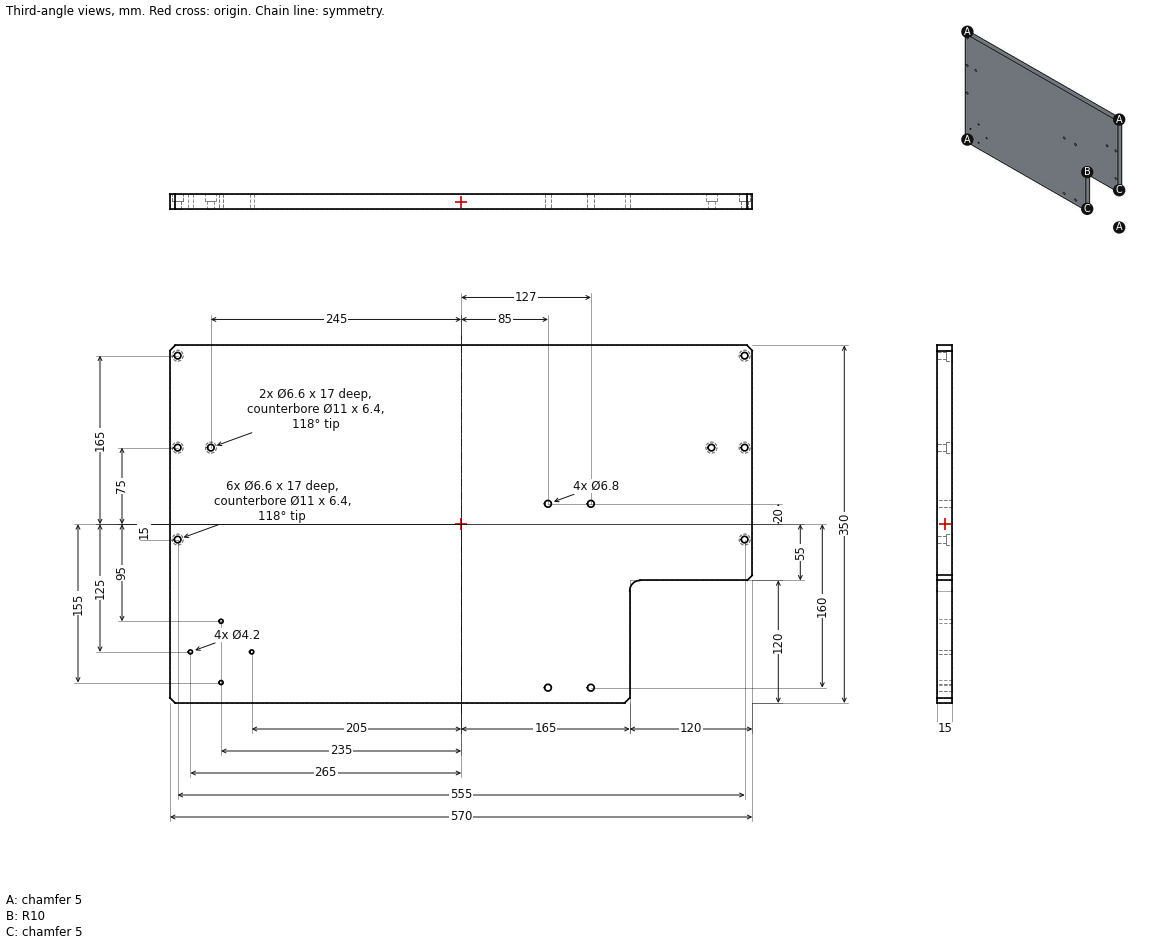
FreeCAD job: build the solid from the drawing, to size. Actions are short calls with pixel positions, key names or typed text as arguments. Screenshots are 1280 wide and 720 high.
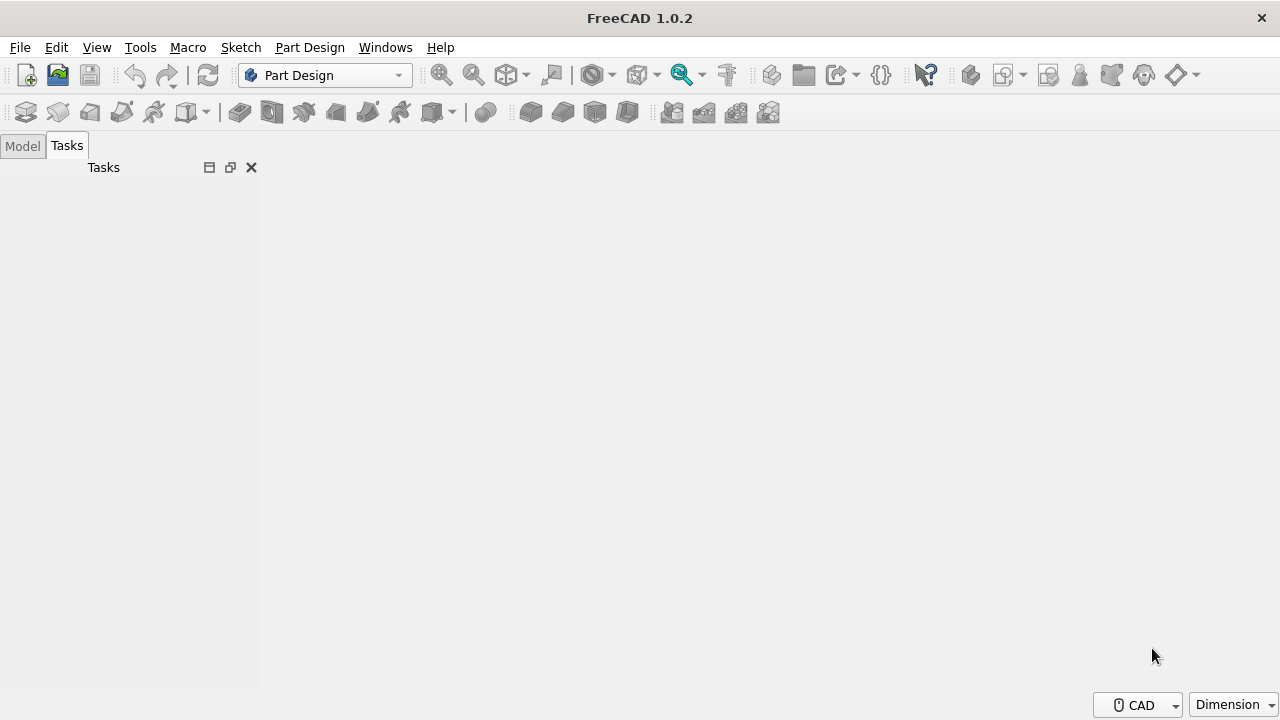
click(26, 76)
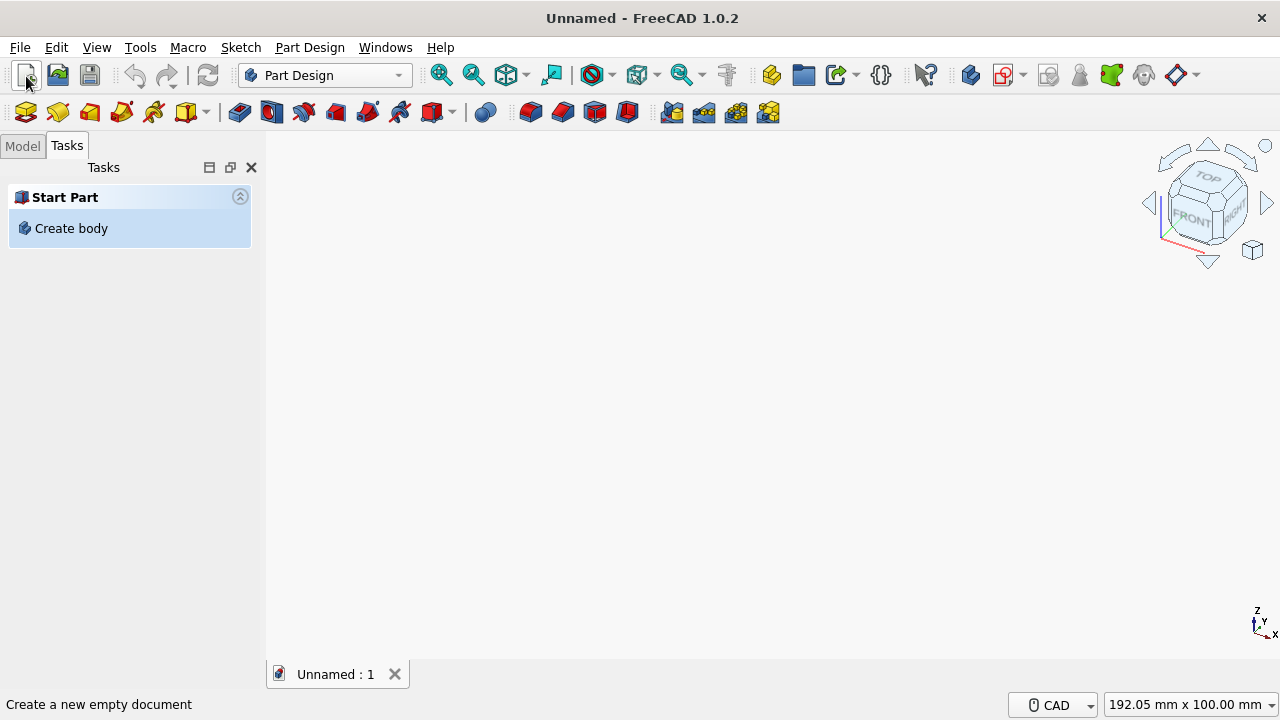
click(1004, 76)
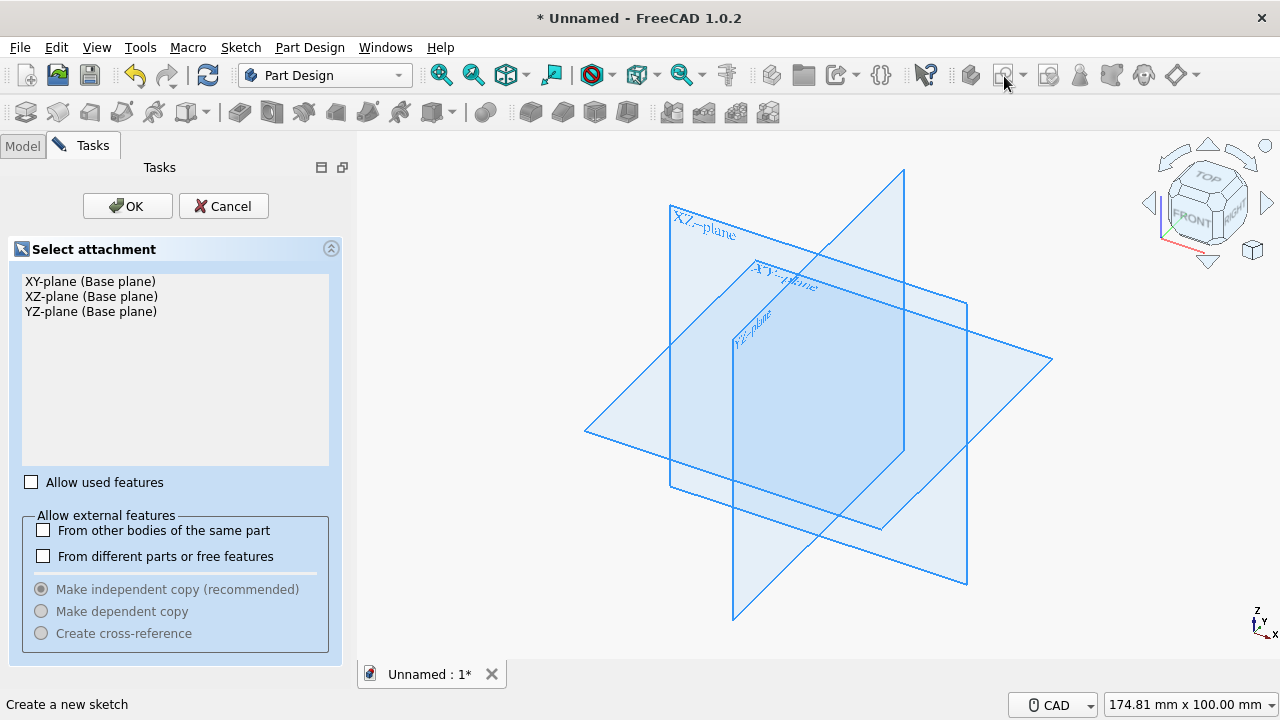
click(82, 296)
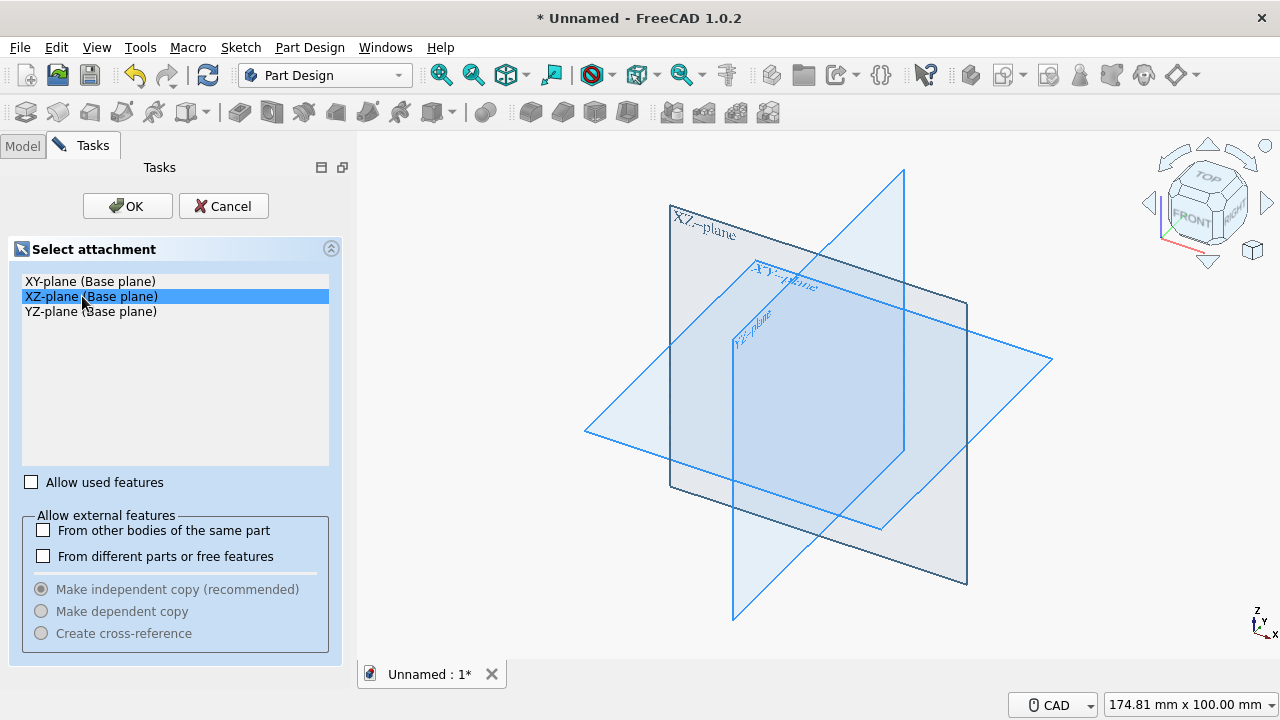
click(128, 206)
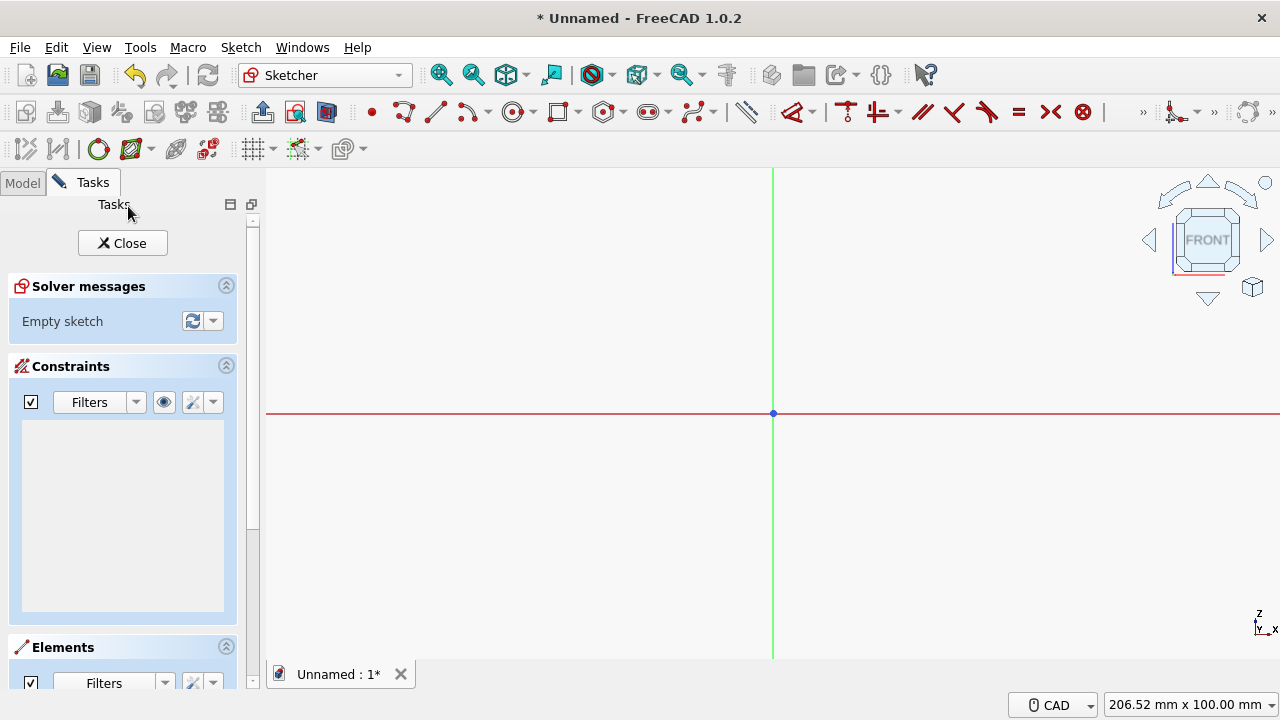
scroll(691, 414, down, 9)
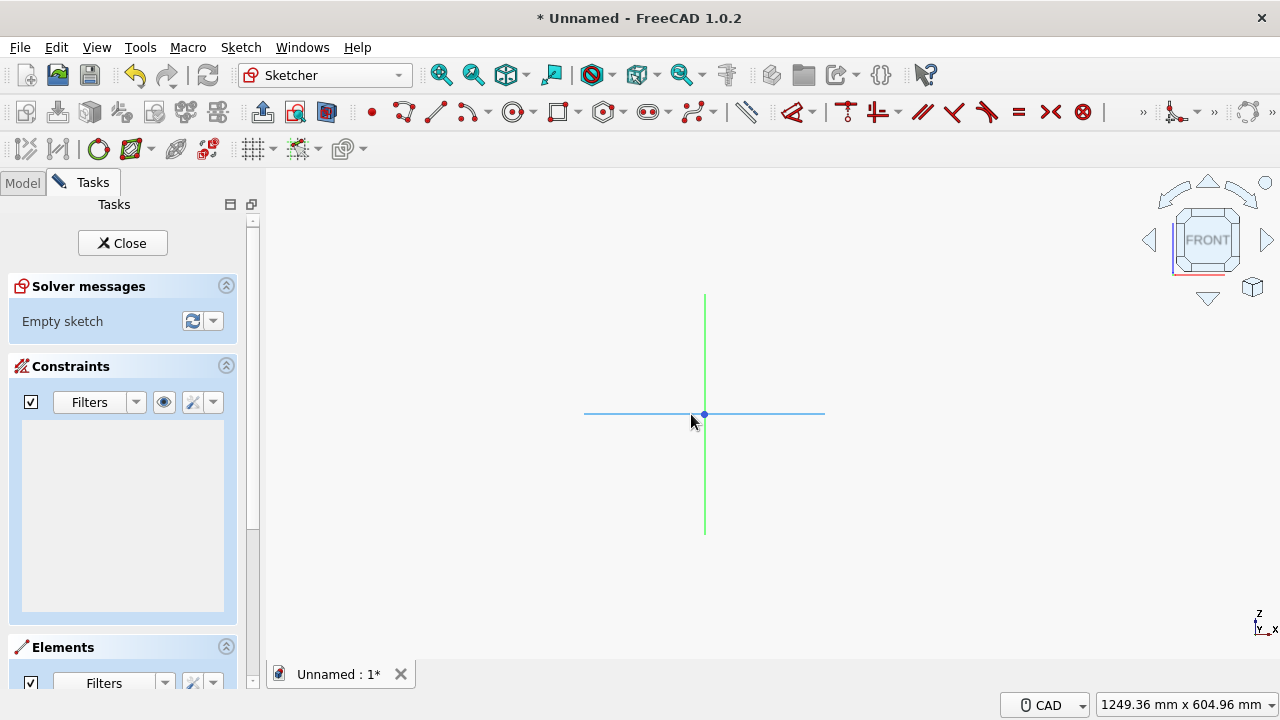
click(580, 112)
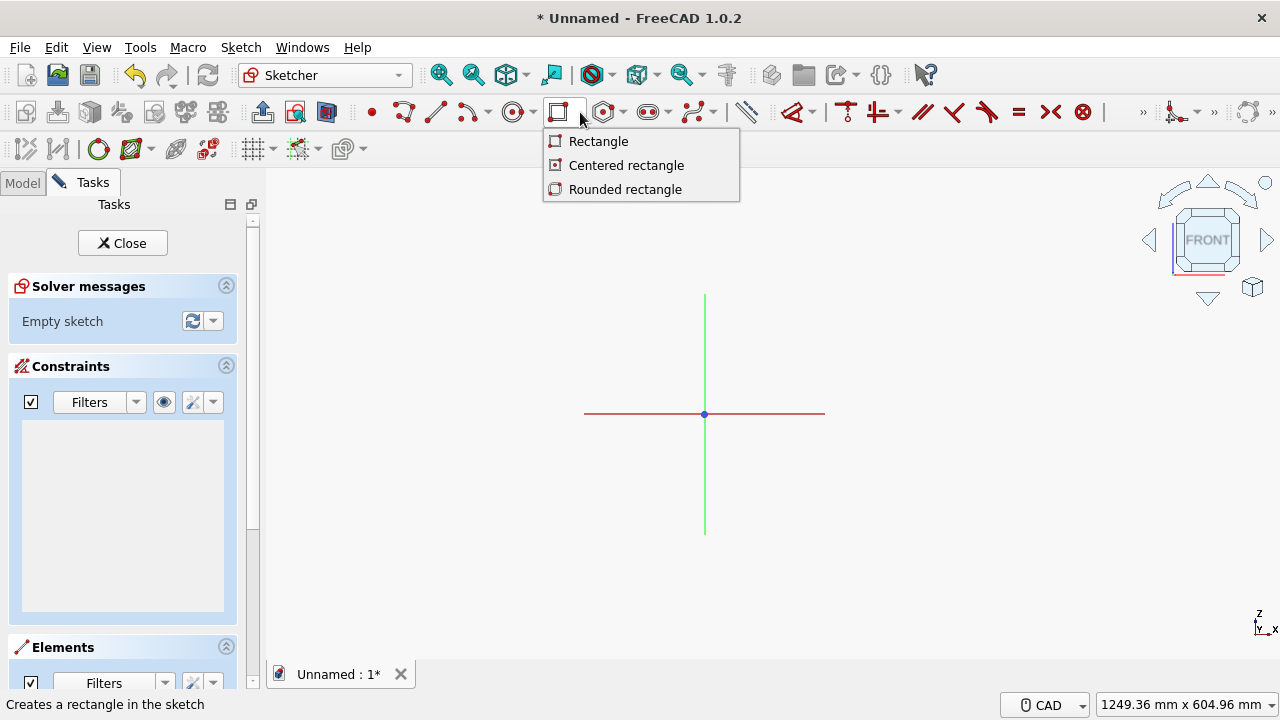
click(642, 165)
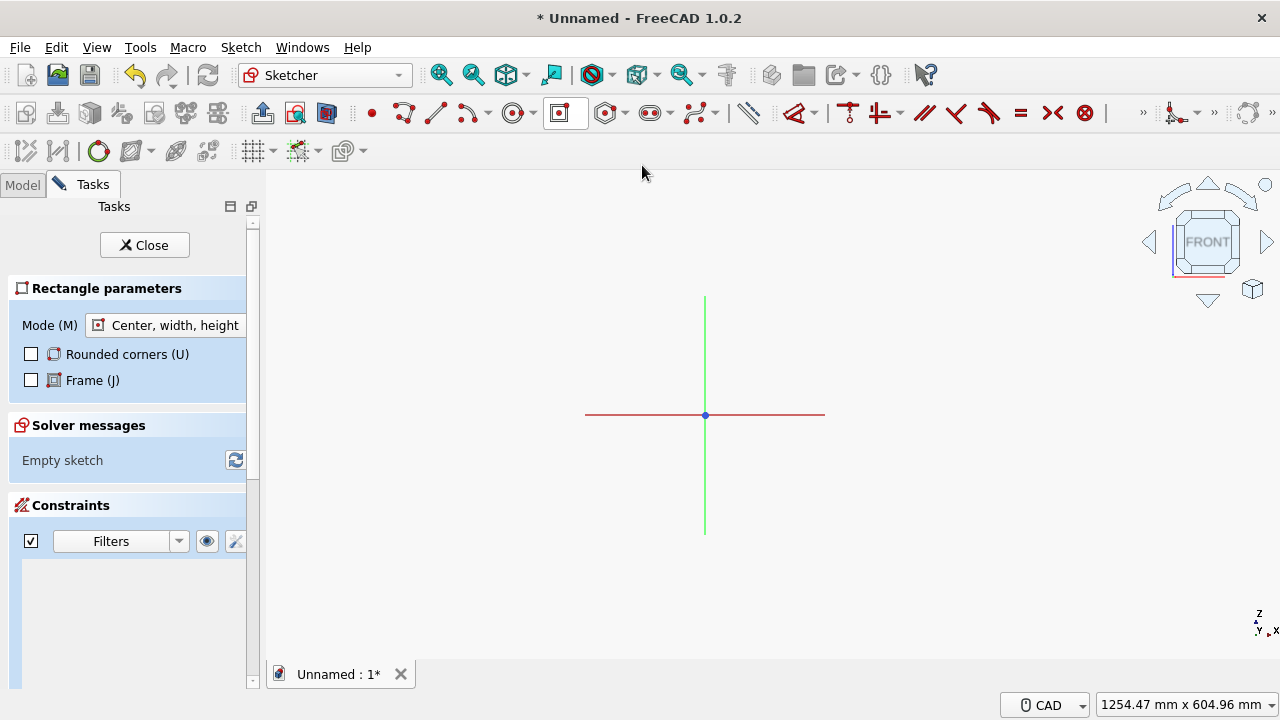
click(705, 415)
move(936, 274)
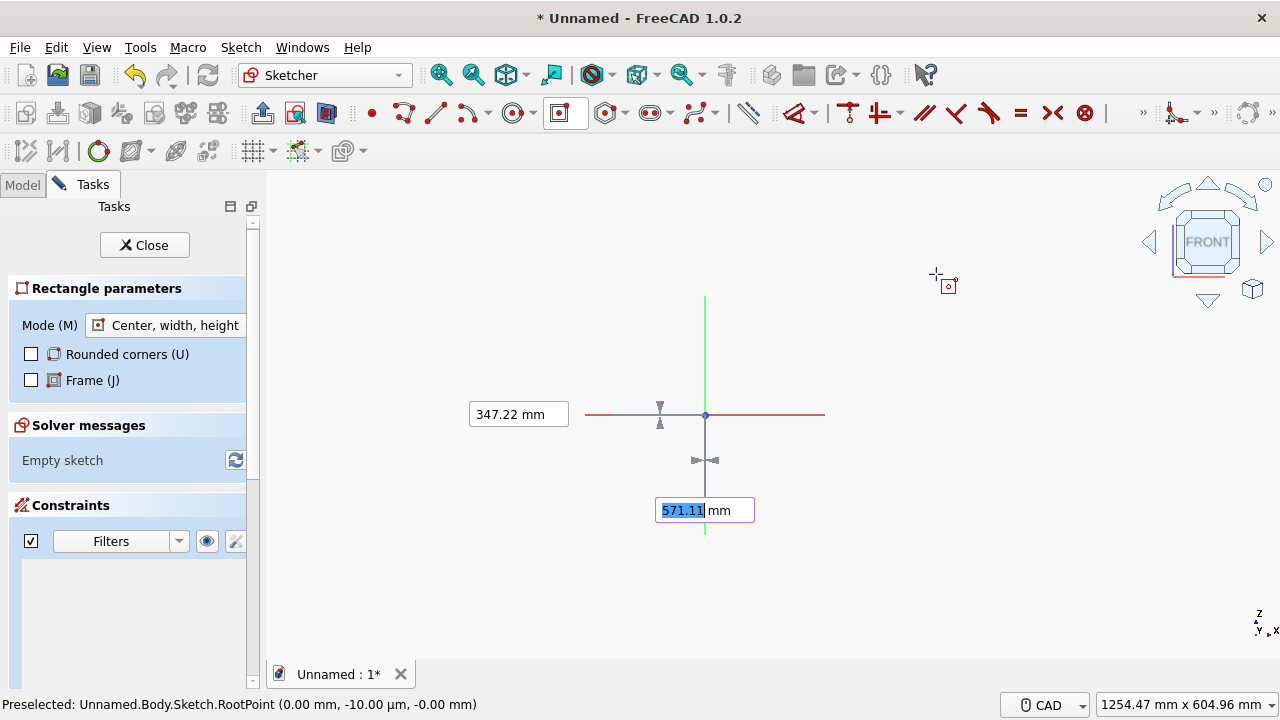
text(570)
key(Tab)
text(350)
key(Return)
key(Escape)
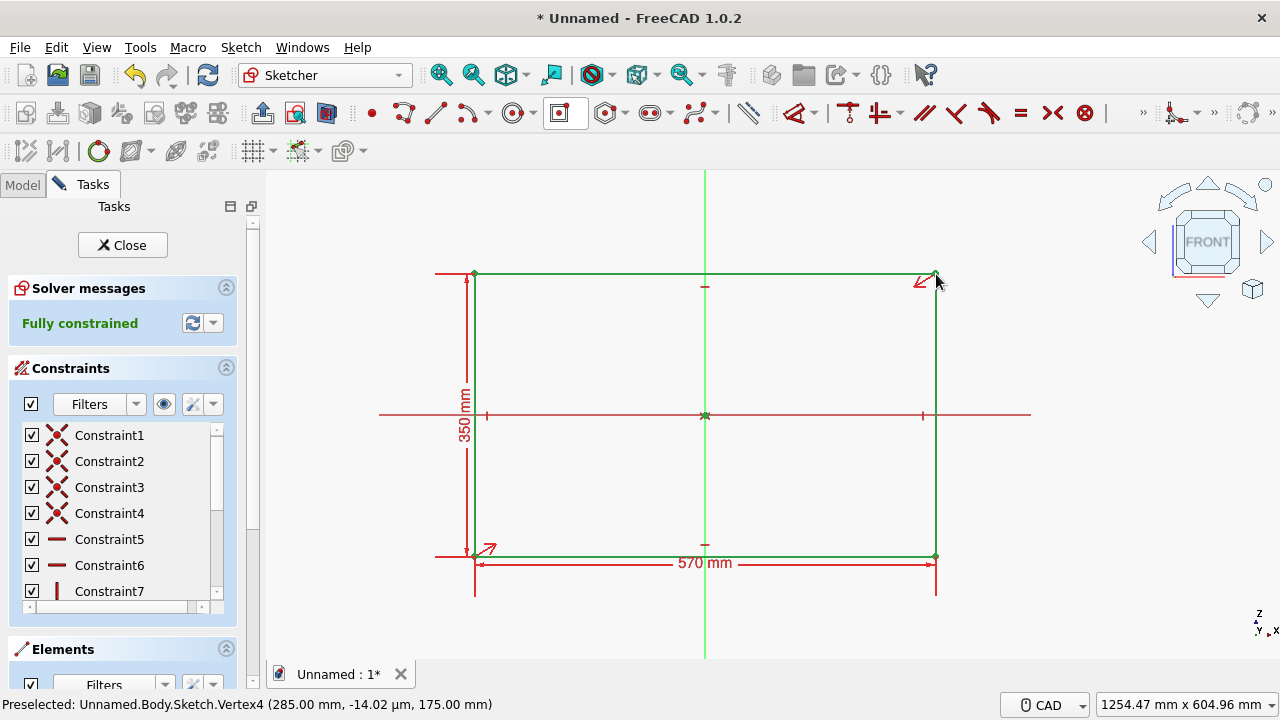
click(123, 245)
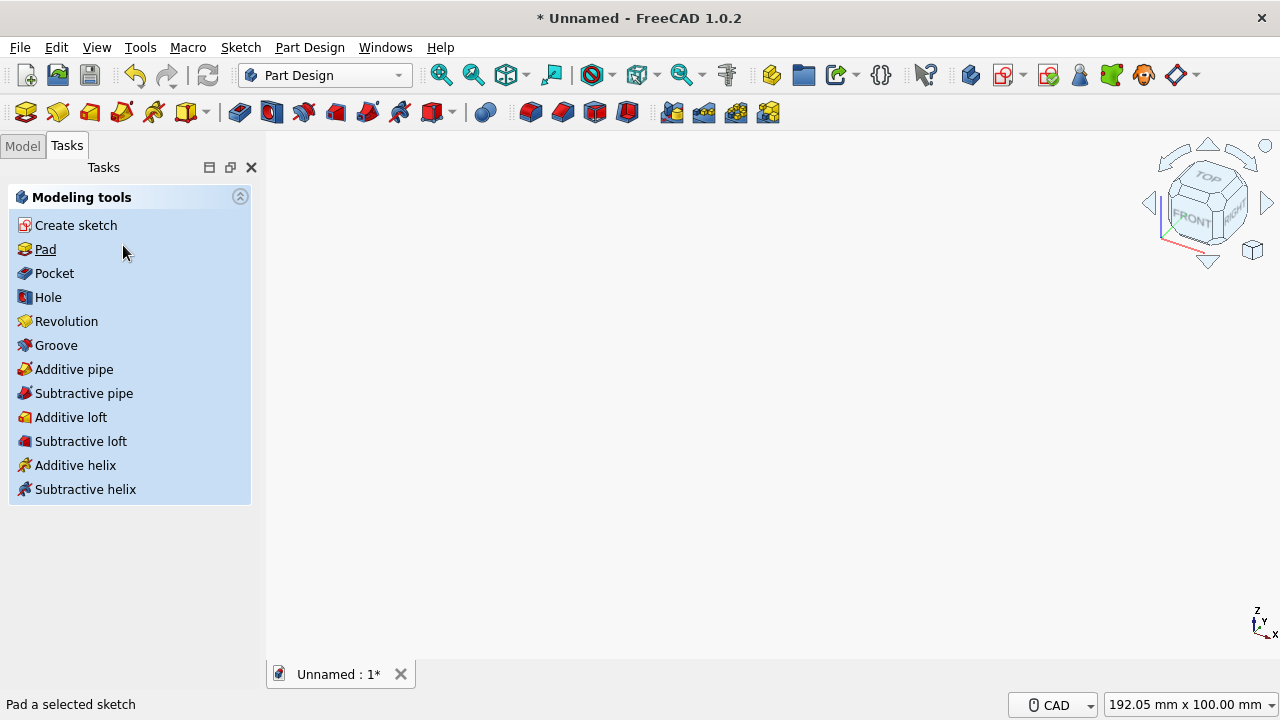
click(26, 112)